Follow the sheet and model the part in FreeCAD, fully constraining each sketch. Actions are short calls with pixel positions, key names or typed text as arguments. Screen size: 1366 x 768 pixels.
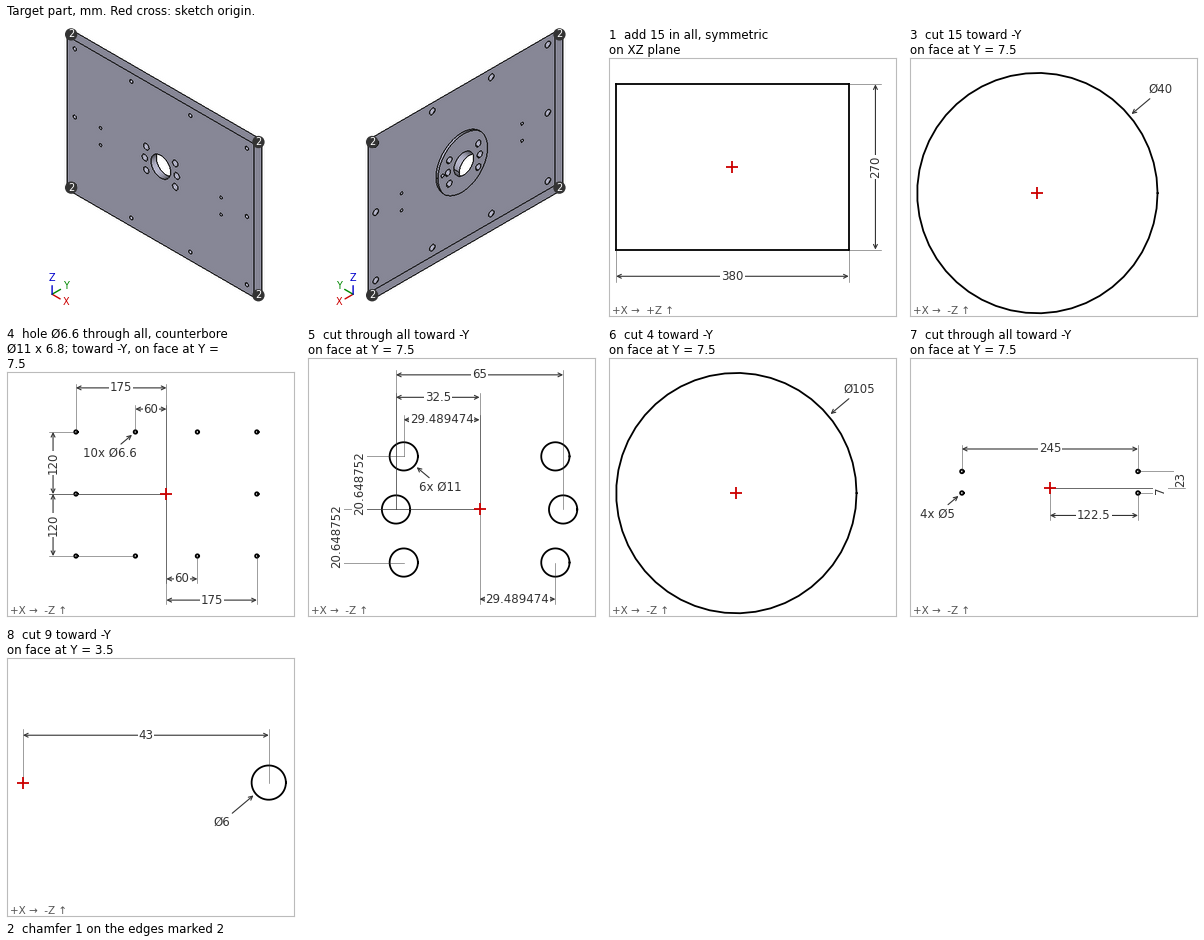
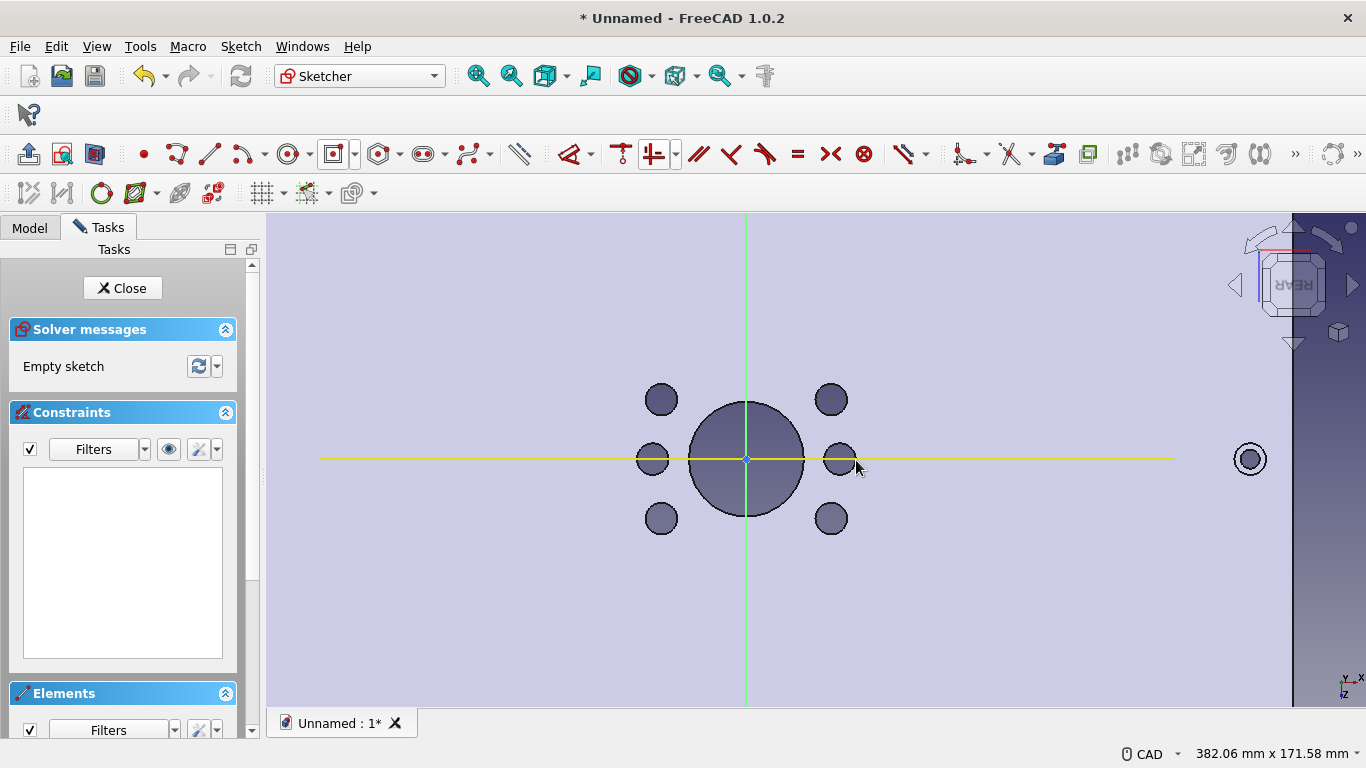
click(288, 154)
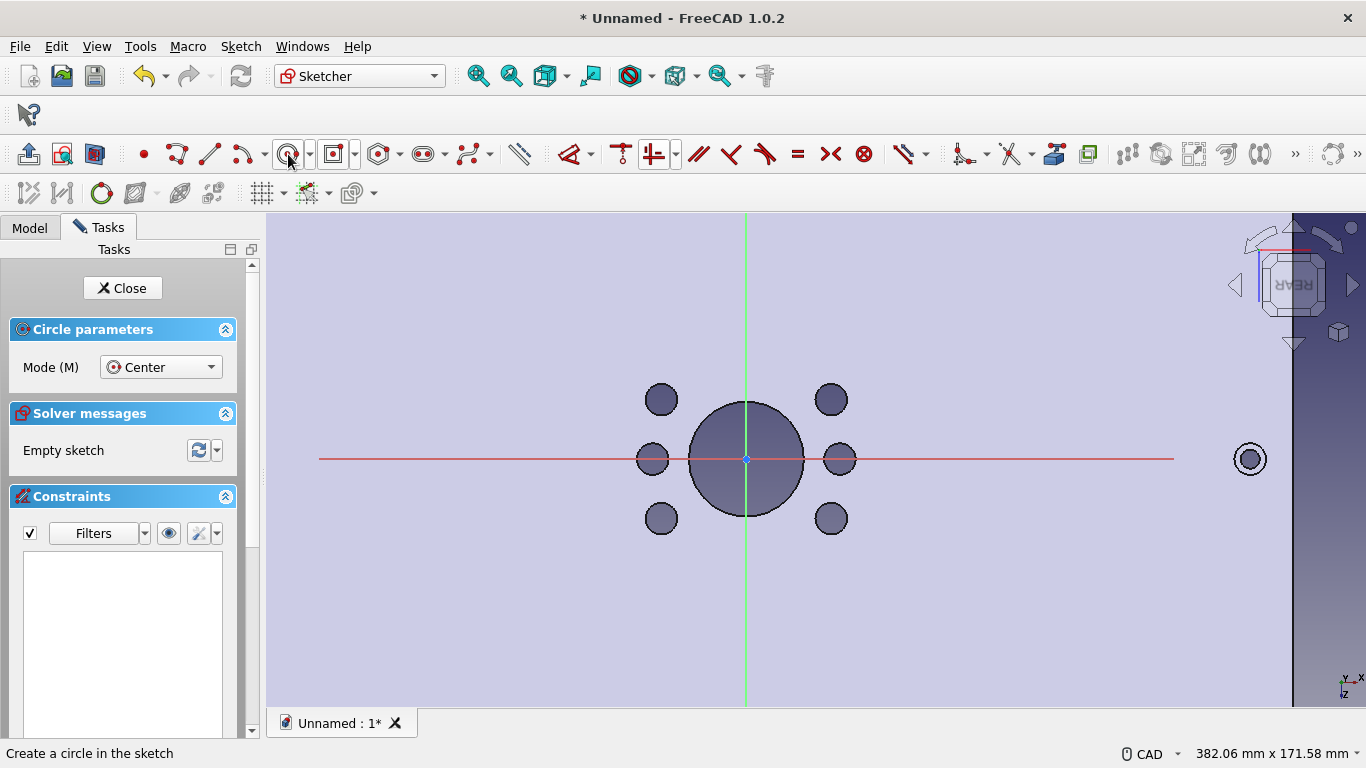
click(746, 459)
click(853, 352)
key(Escape)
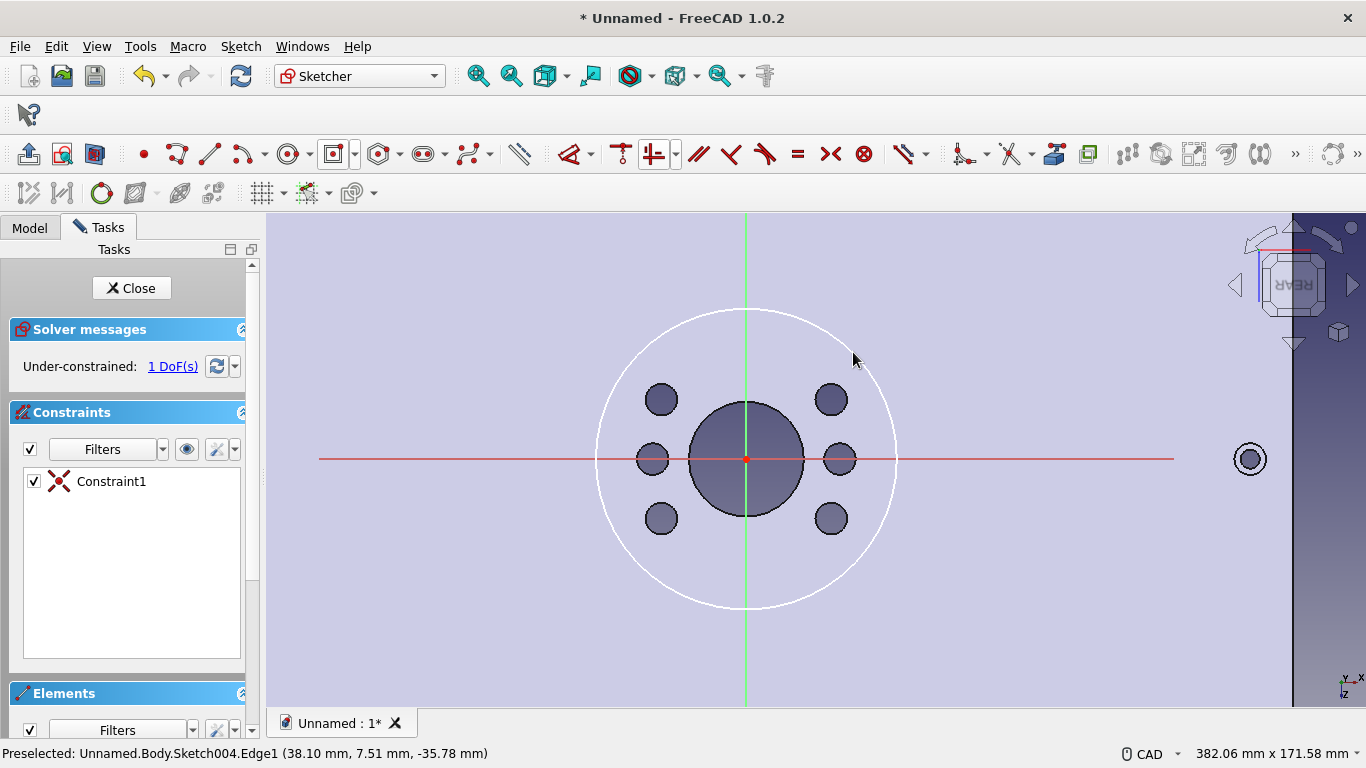
click(568, 154)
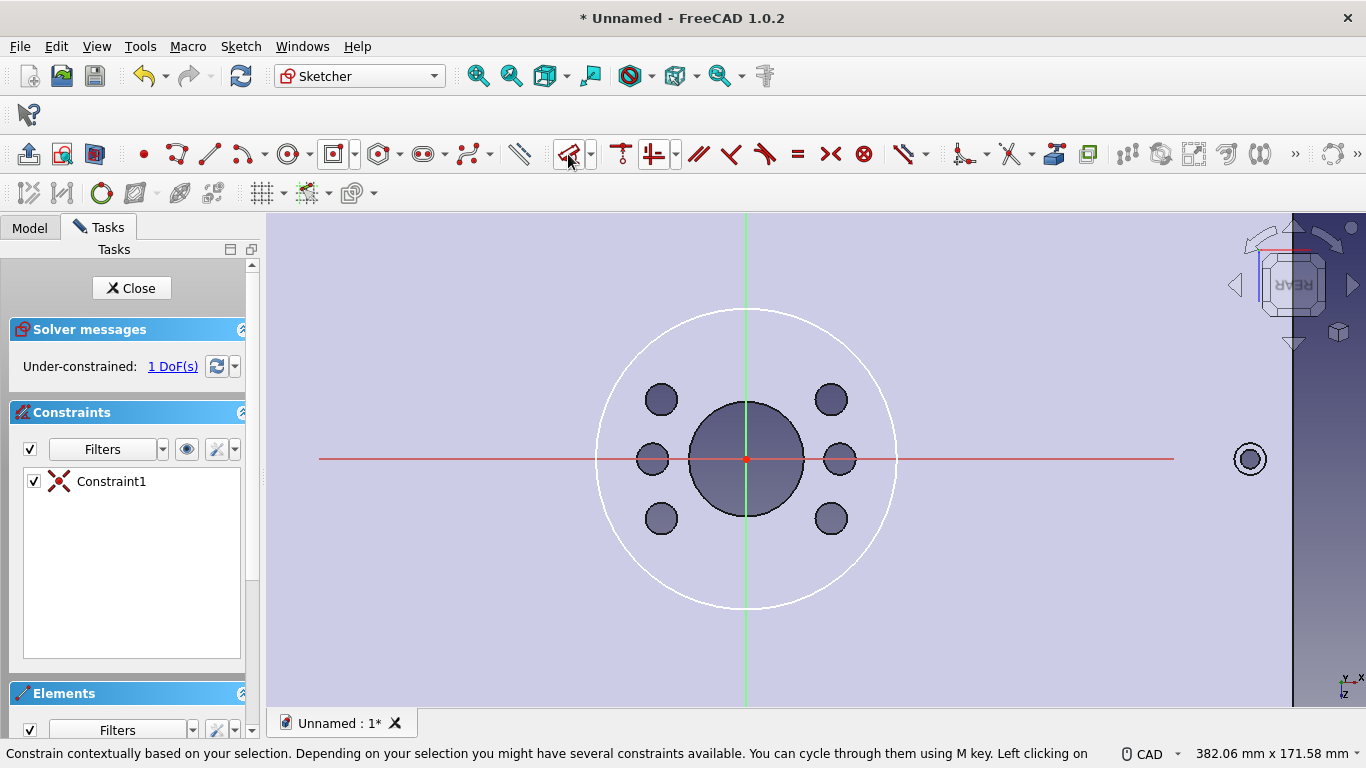
click(852, 352)
click(874, 329)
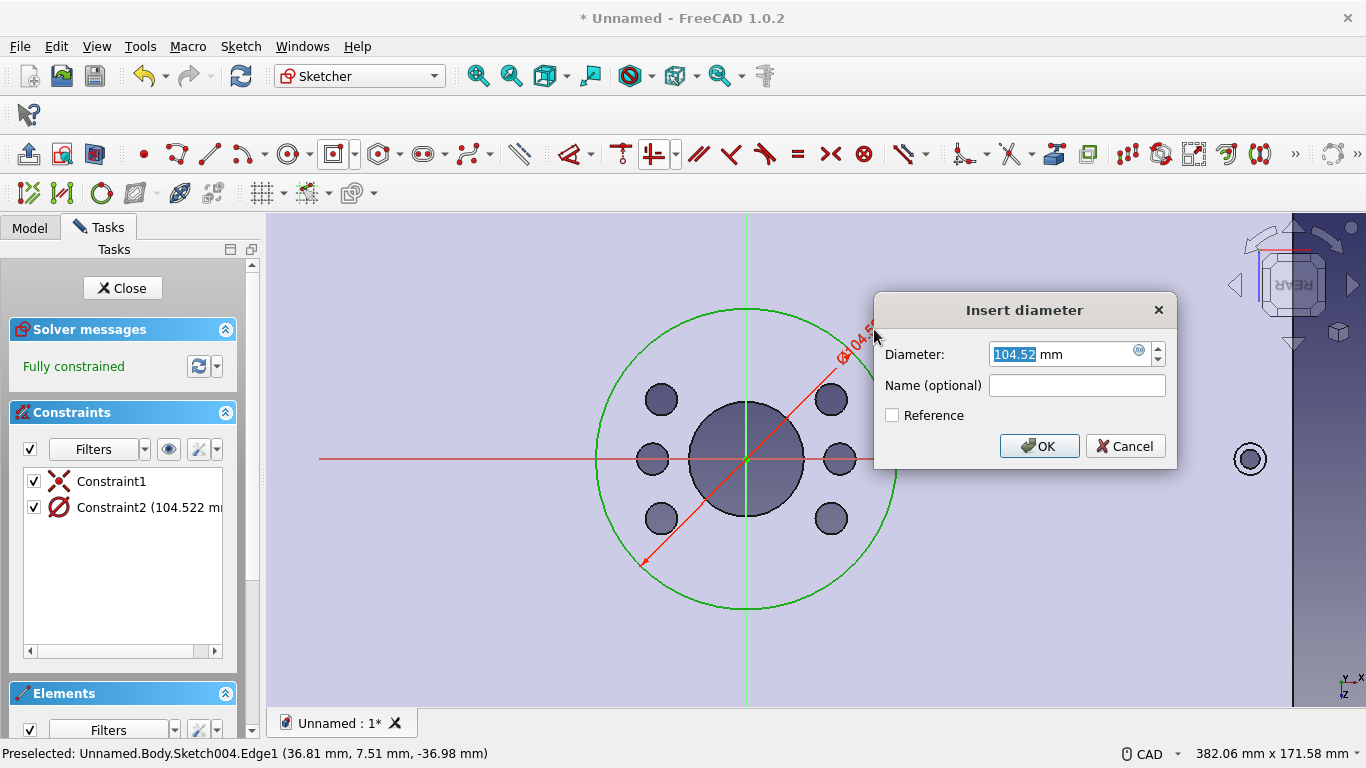
text(105)
key(Return)
key(Escape)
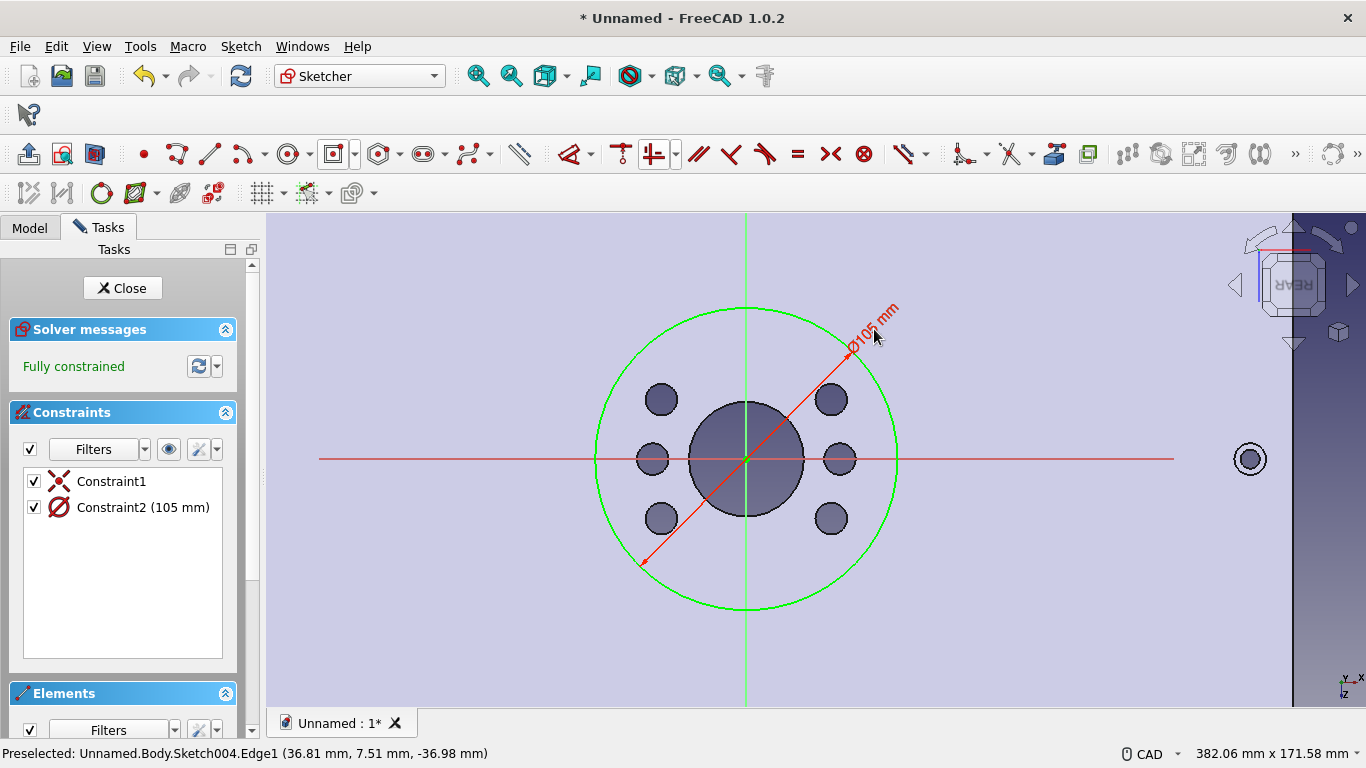
click(123, 288)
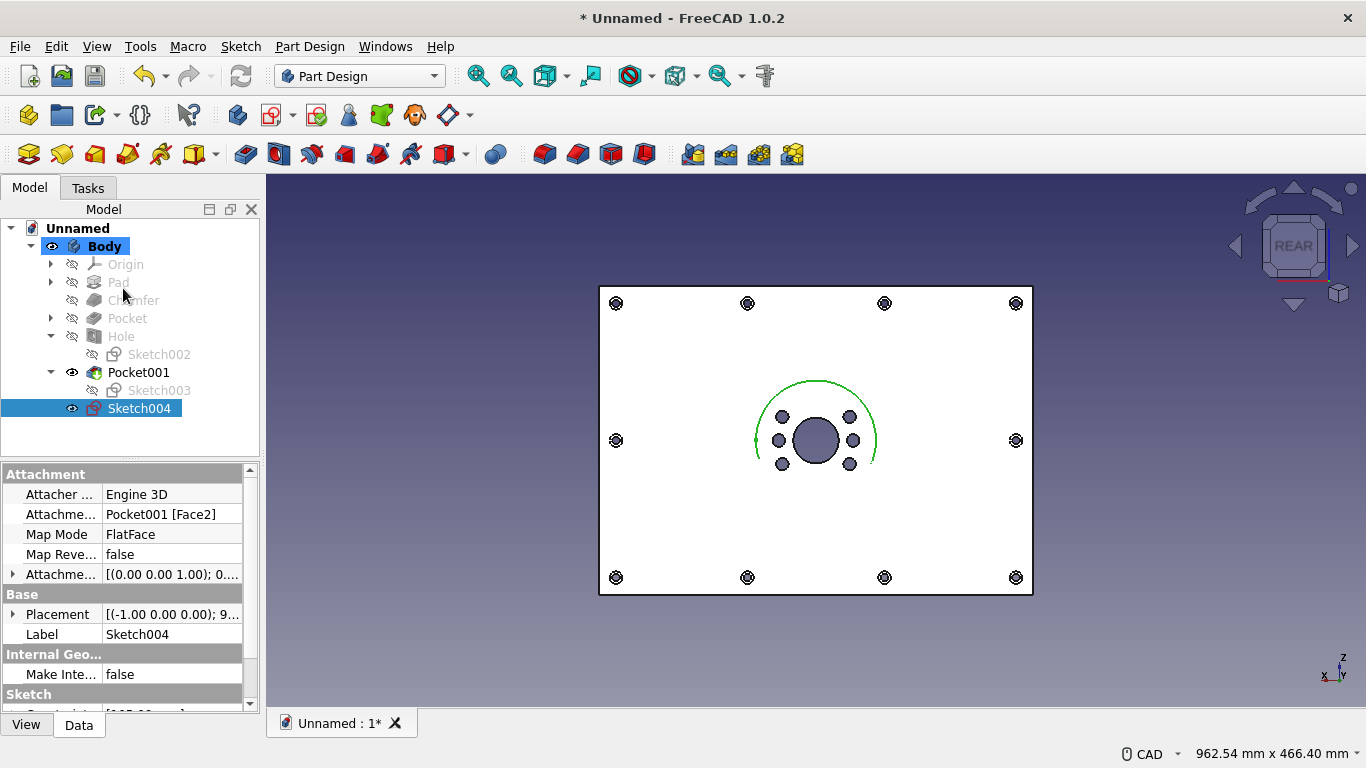
click(246, 154)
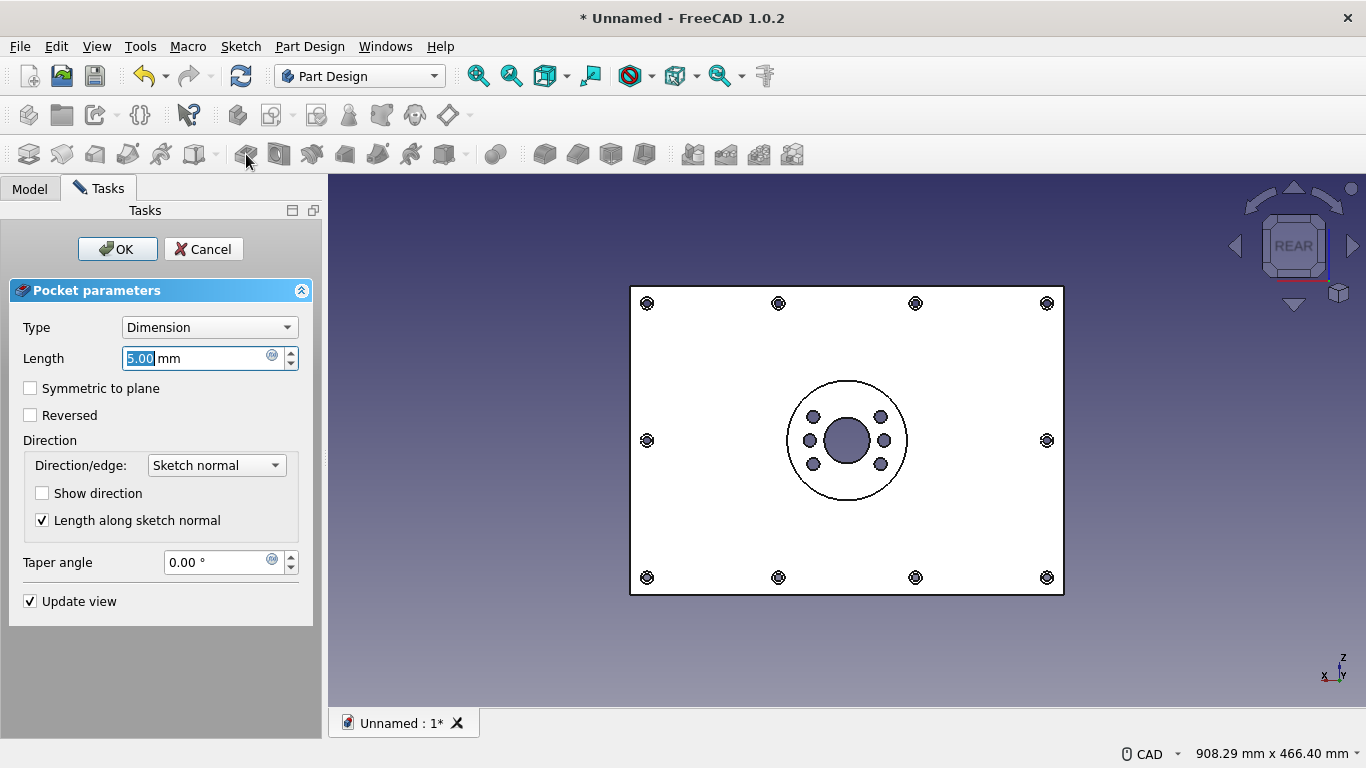
text(4)
key(Tab)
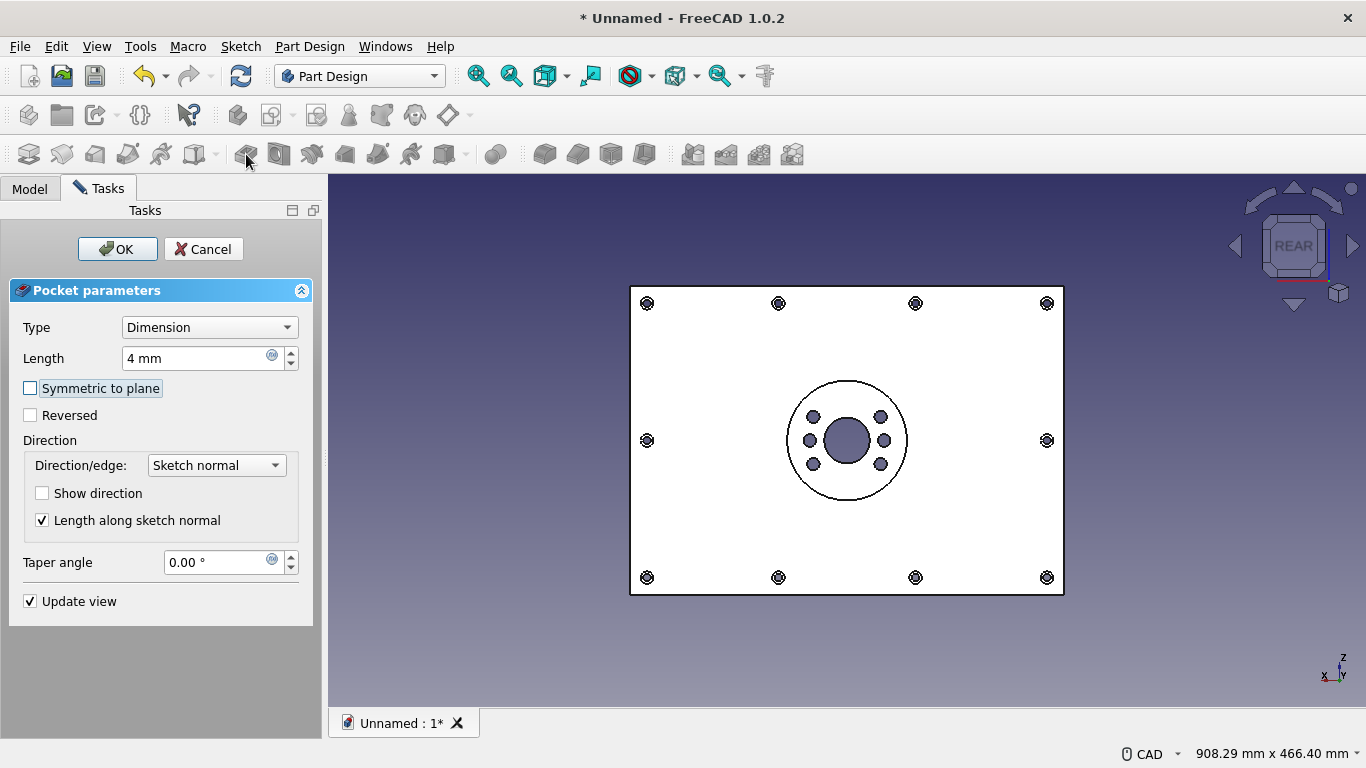
click(118, 249)